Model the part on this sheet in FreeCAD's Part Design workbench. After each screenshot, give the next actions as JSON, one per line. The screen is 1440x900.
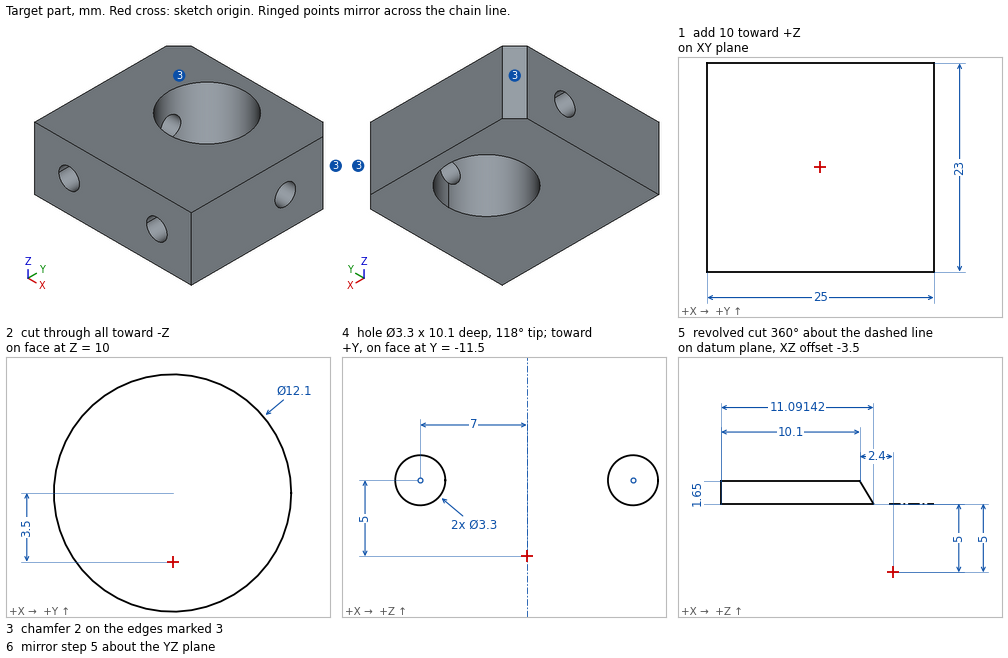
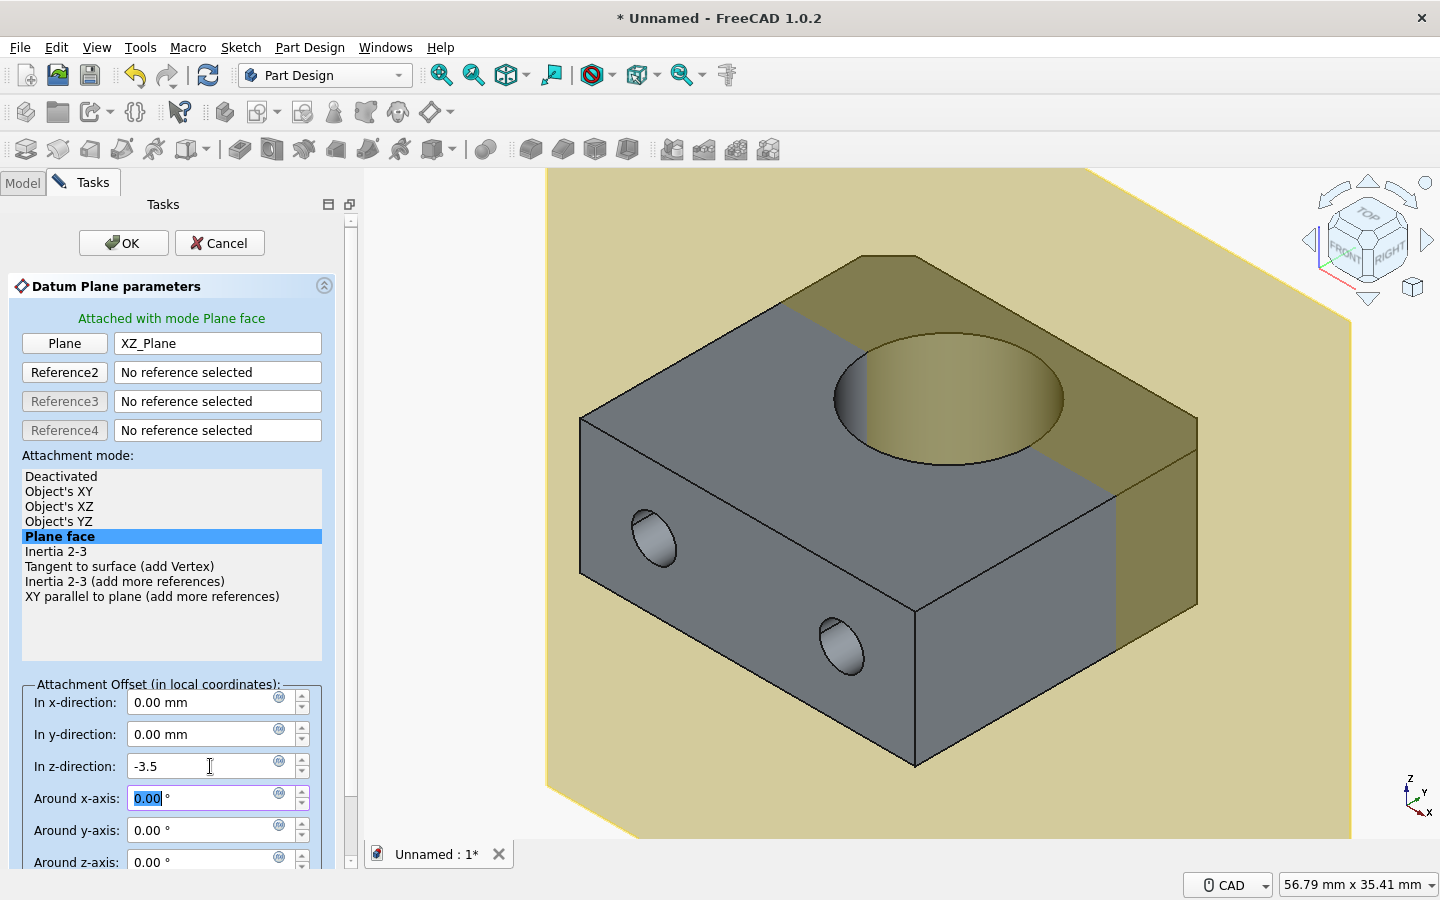
{"action": "left_click", "coordinate": [124, 243]}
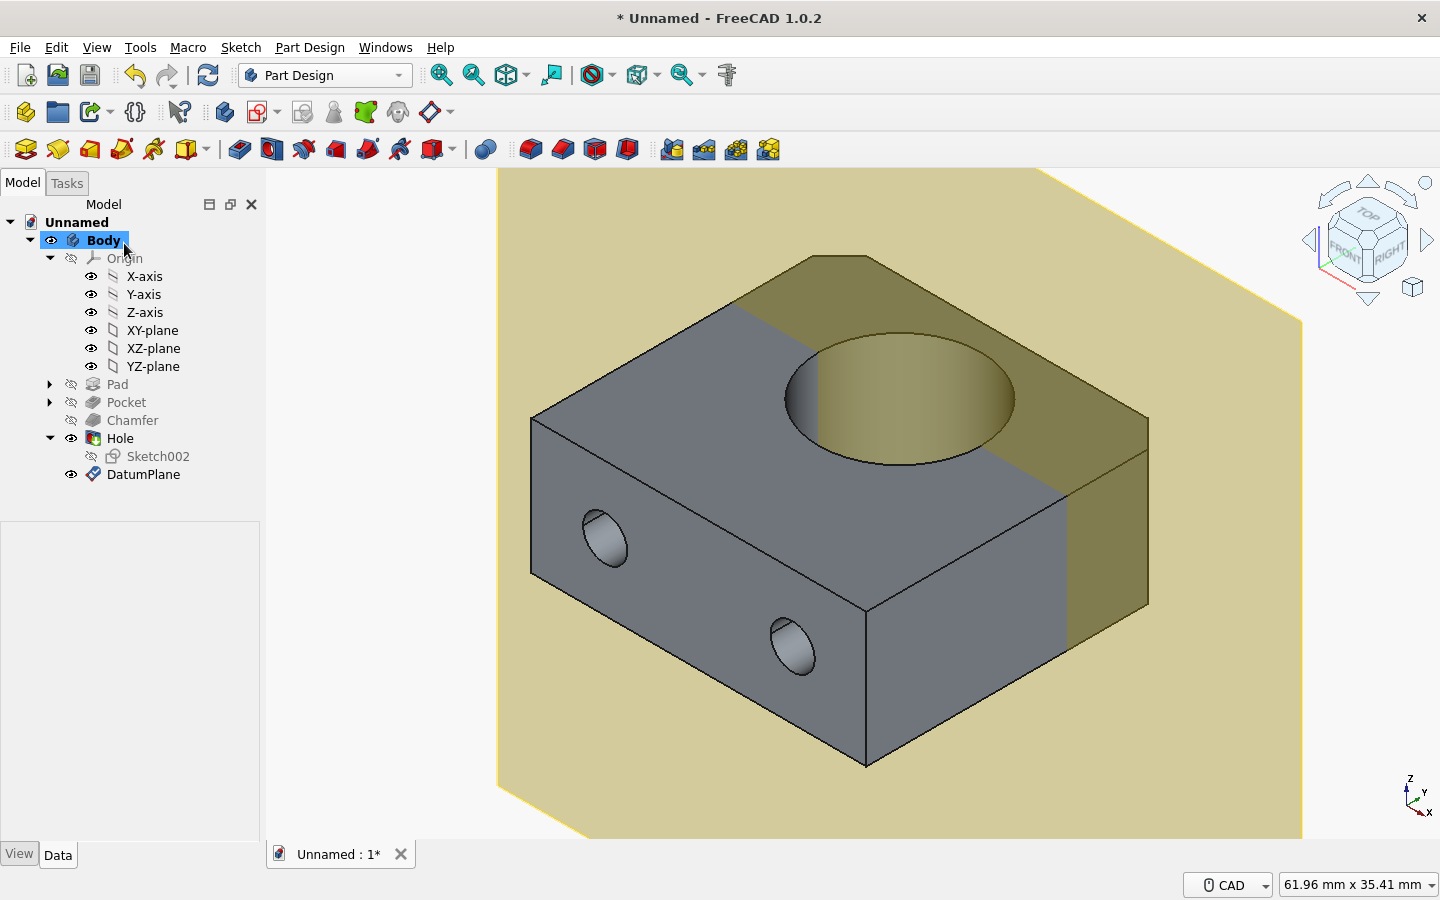
{"action": "left_click", "coordinate": [116, 474]}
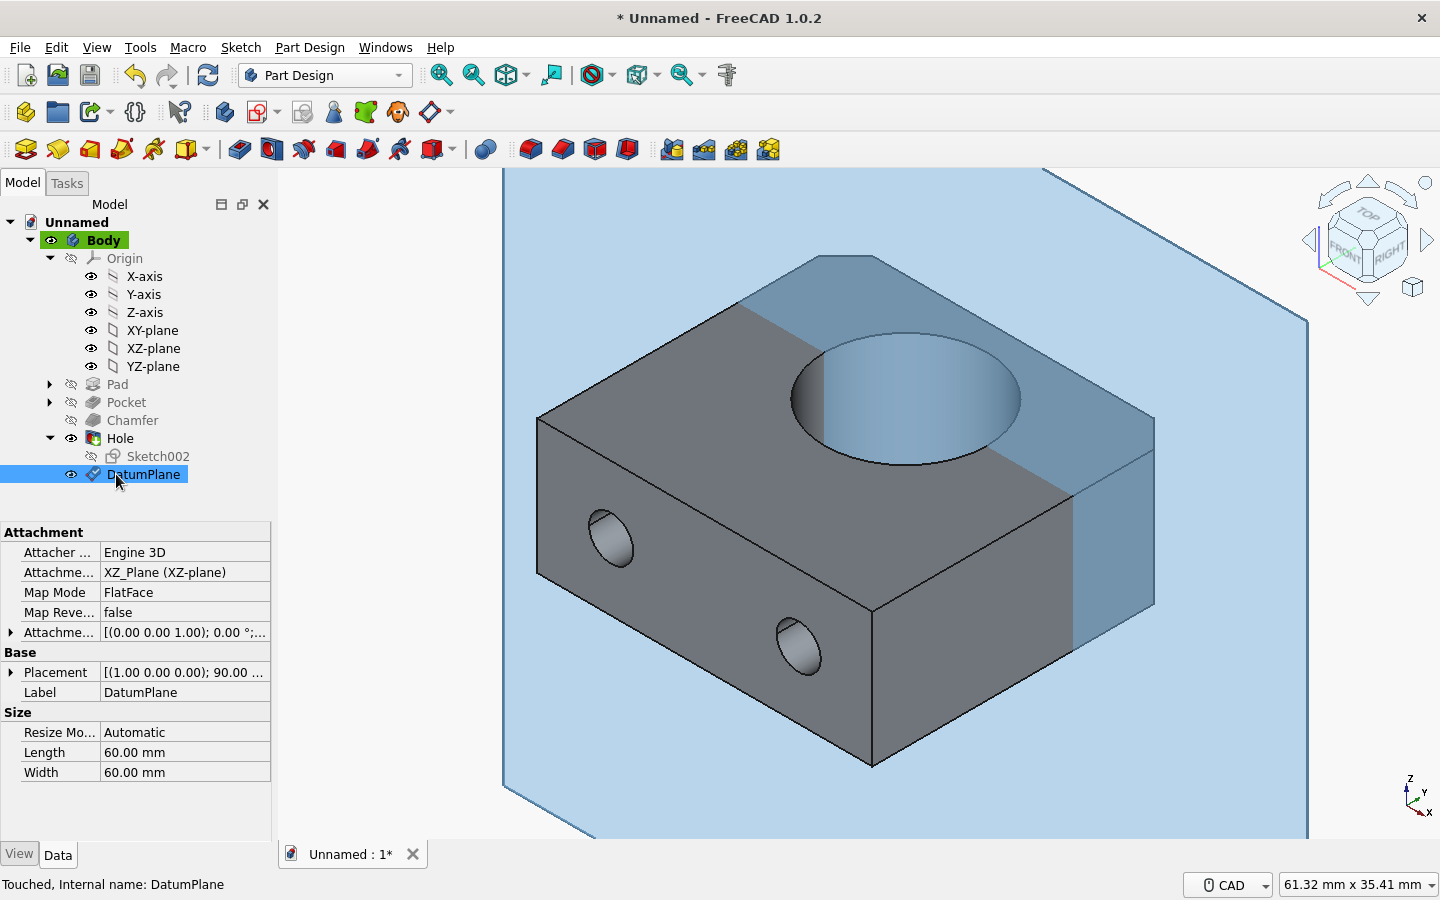
{"action": "left_click", "coordinate": [258, 112]}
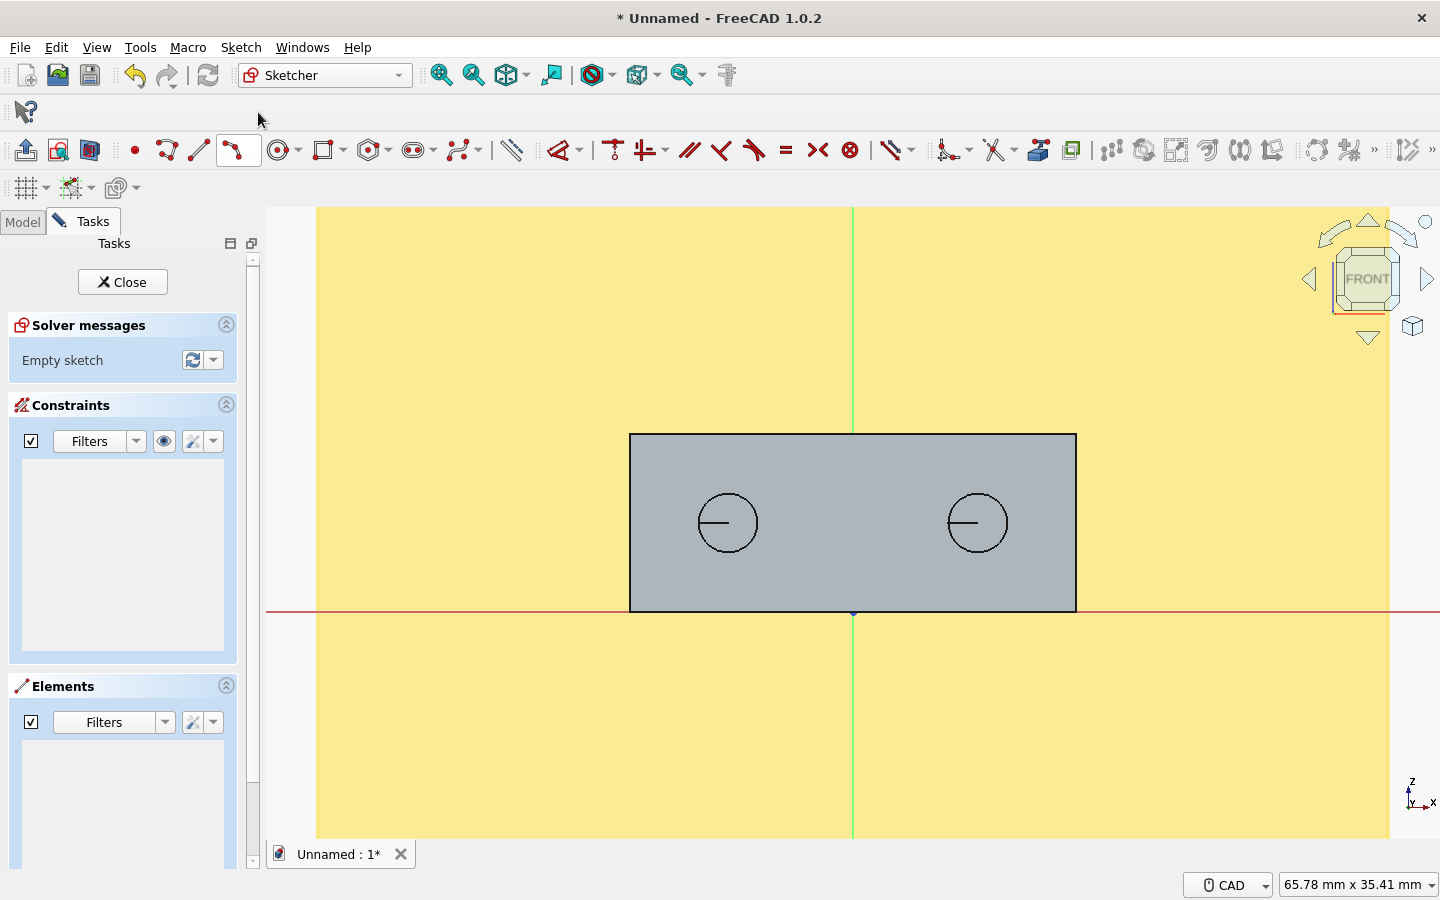
{"action": "left_click", "coordinate": [90, 150]}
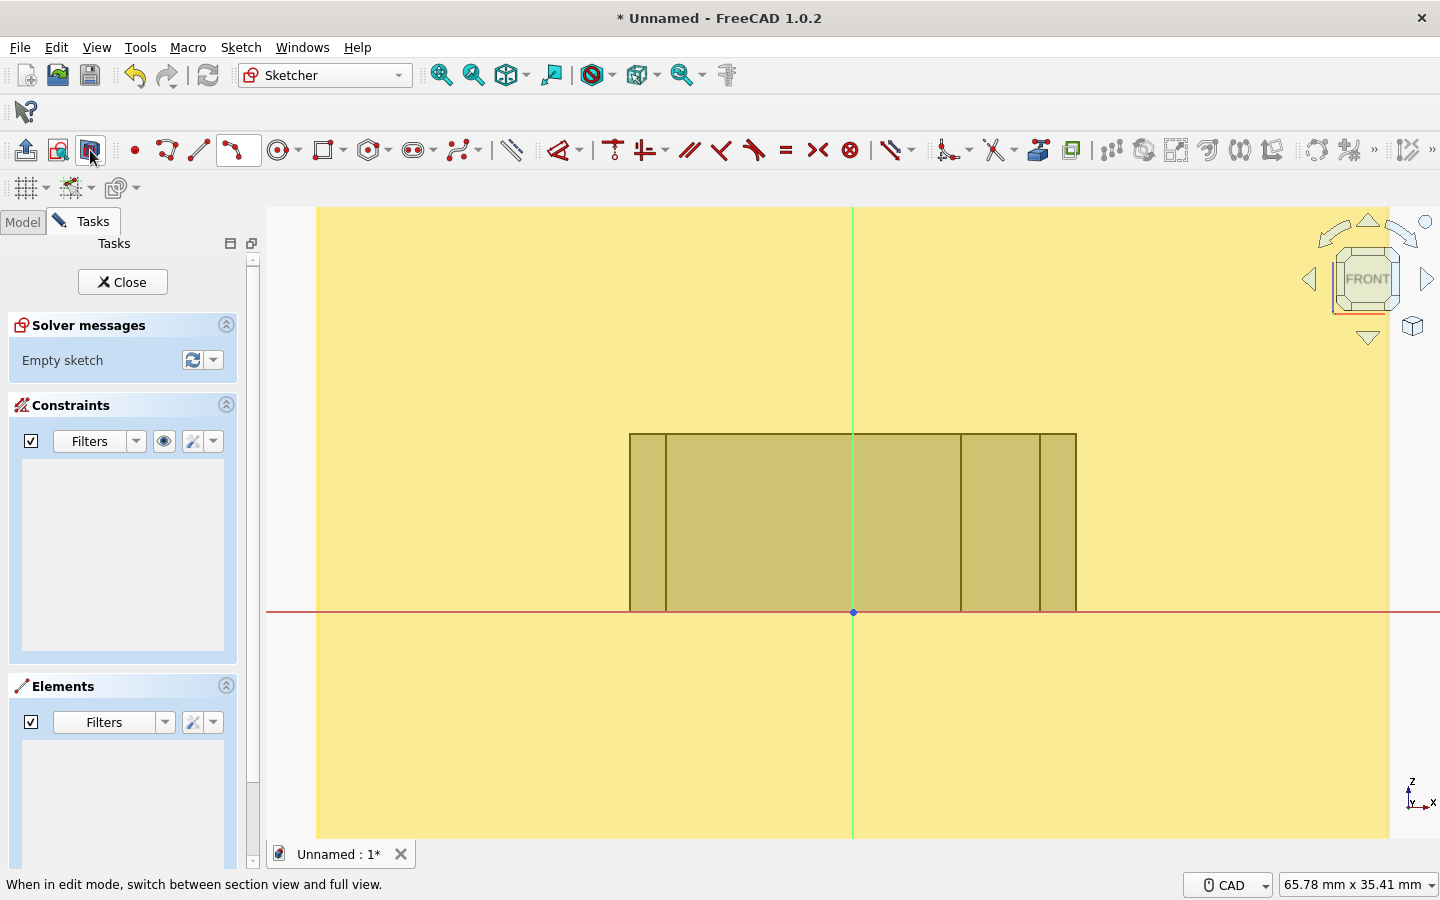
{"action": "scroll", "coordinate": [759, 570], "scroll_direction": "up", "scroll_amount": 5}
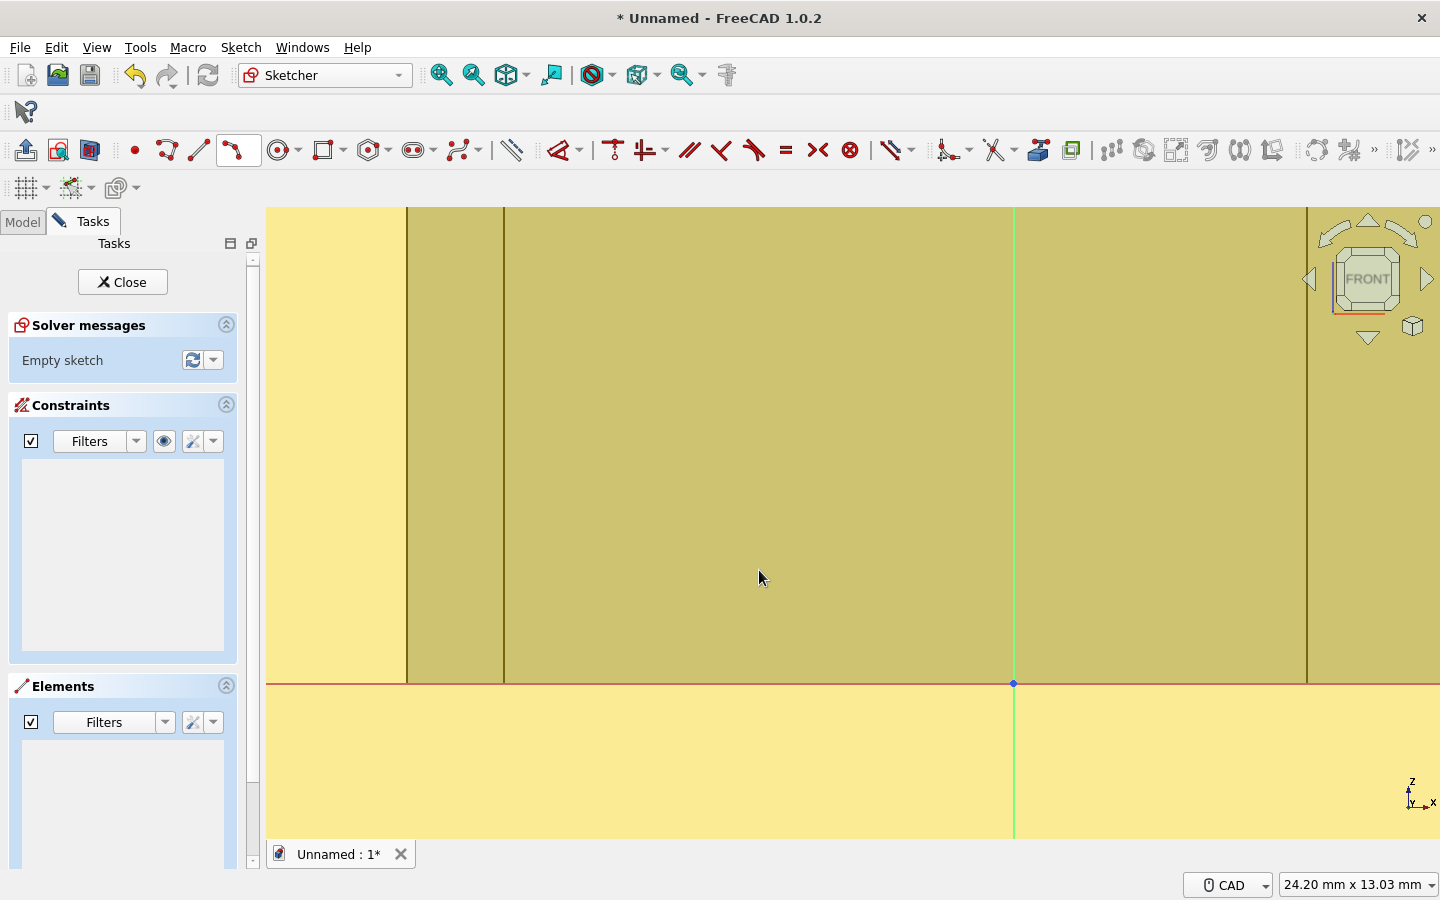
{"action": "left_click", "coordinate": [168, 150]}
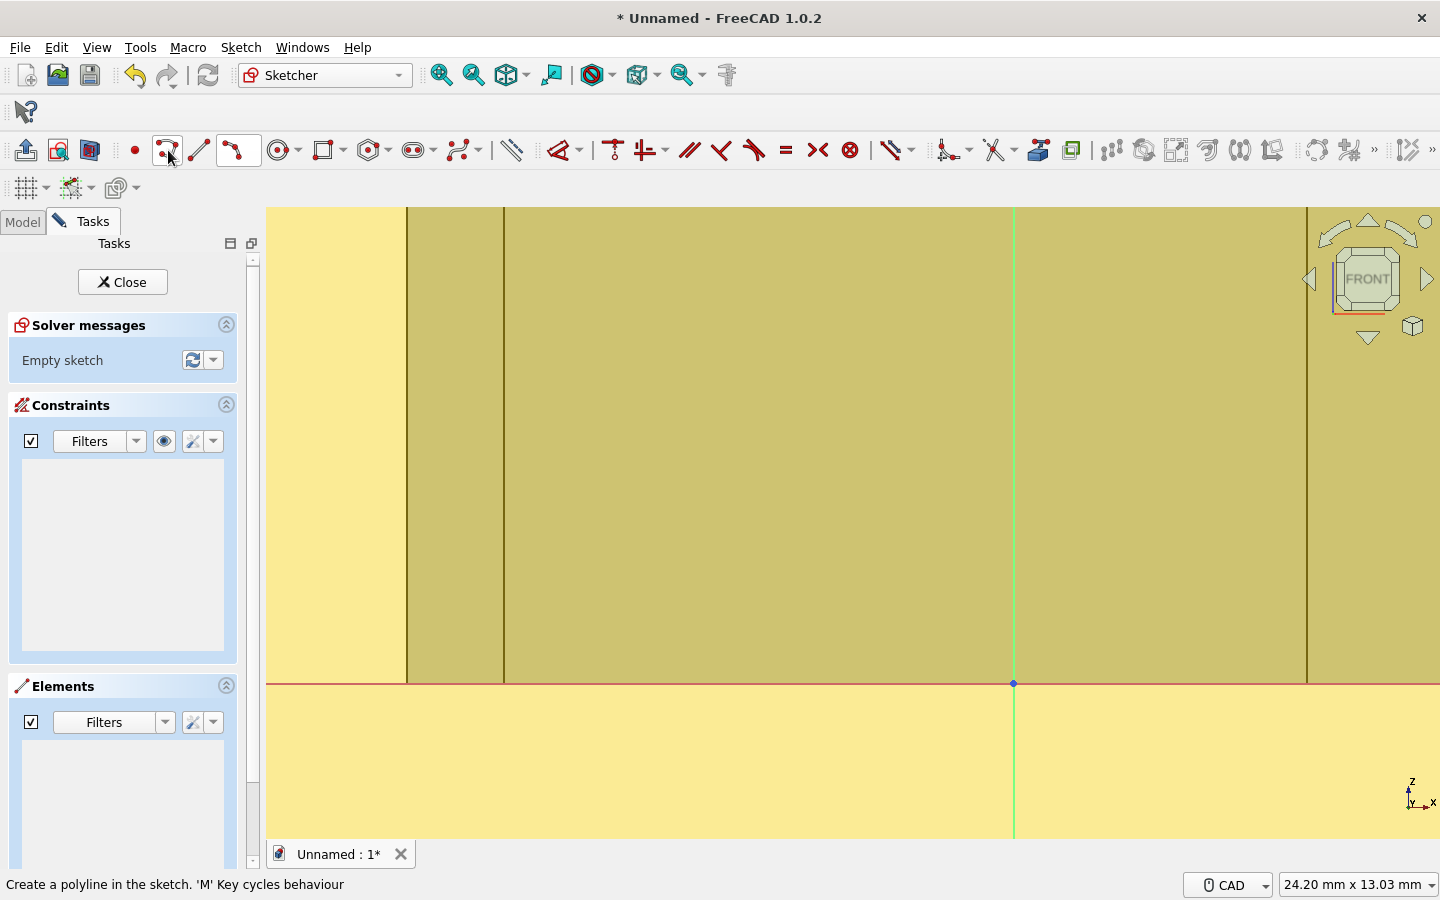
{"action": "left_click", "coordinate": [945, 441]}
{"action": "left_click", "coordinate": [407, 441]}
{"action": "left_click", "coordinate": [407, 361]}
{"action": "left_click", "coordinate": [897, 361]}
{"action": "left_click", "coordinate": [945, 442]}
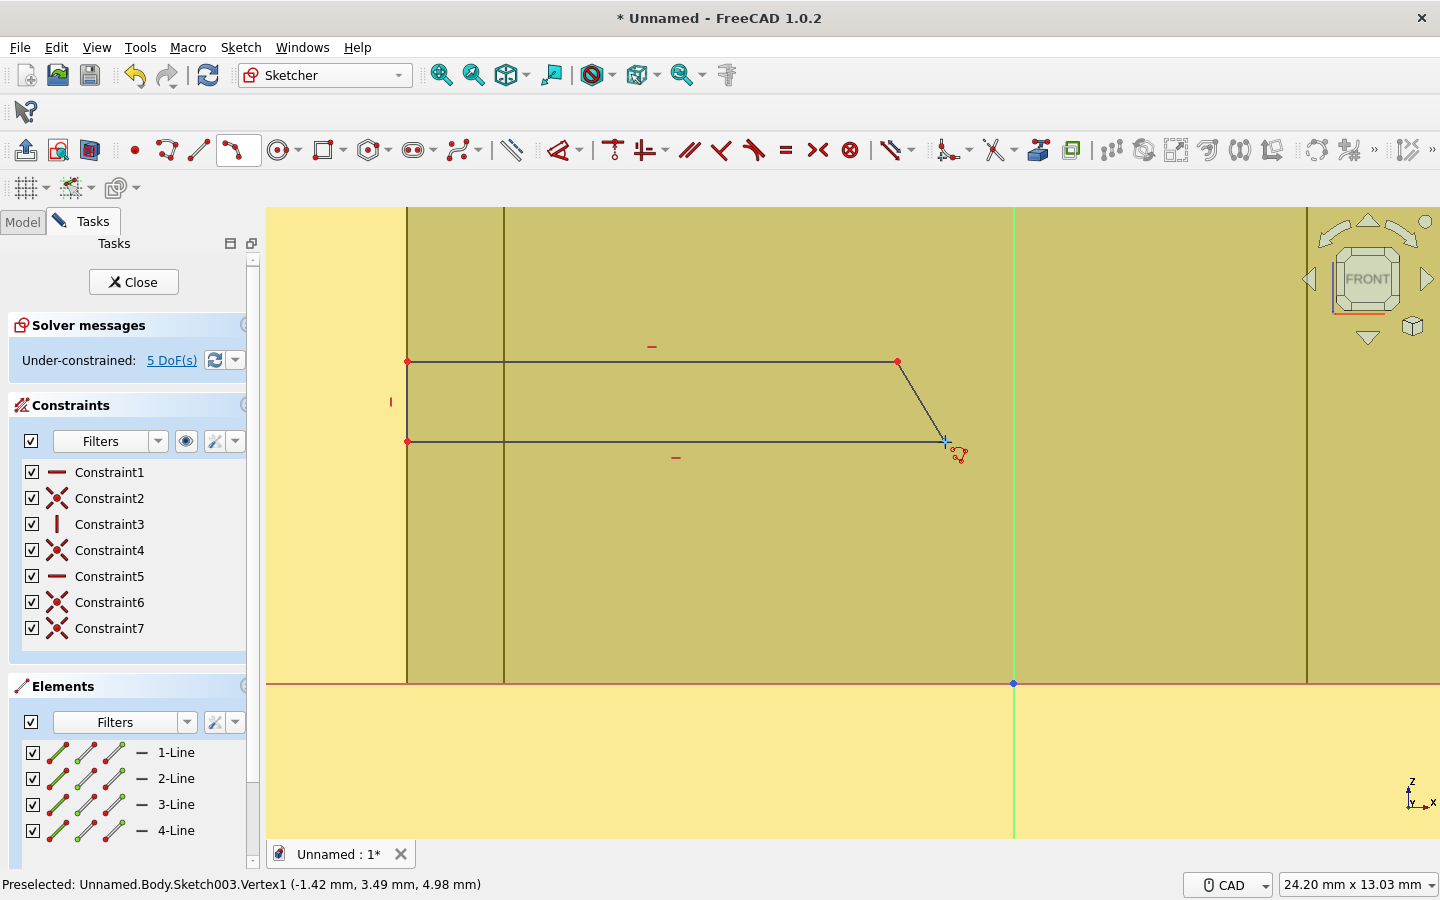
{"action": "left_click", "coordinate": [200, 150]}